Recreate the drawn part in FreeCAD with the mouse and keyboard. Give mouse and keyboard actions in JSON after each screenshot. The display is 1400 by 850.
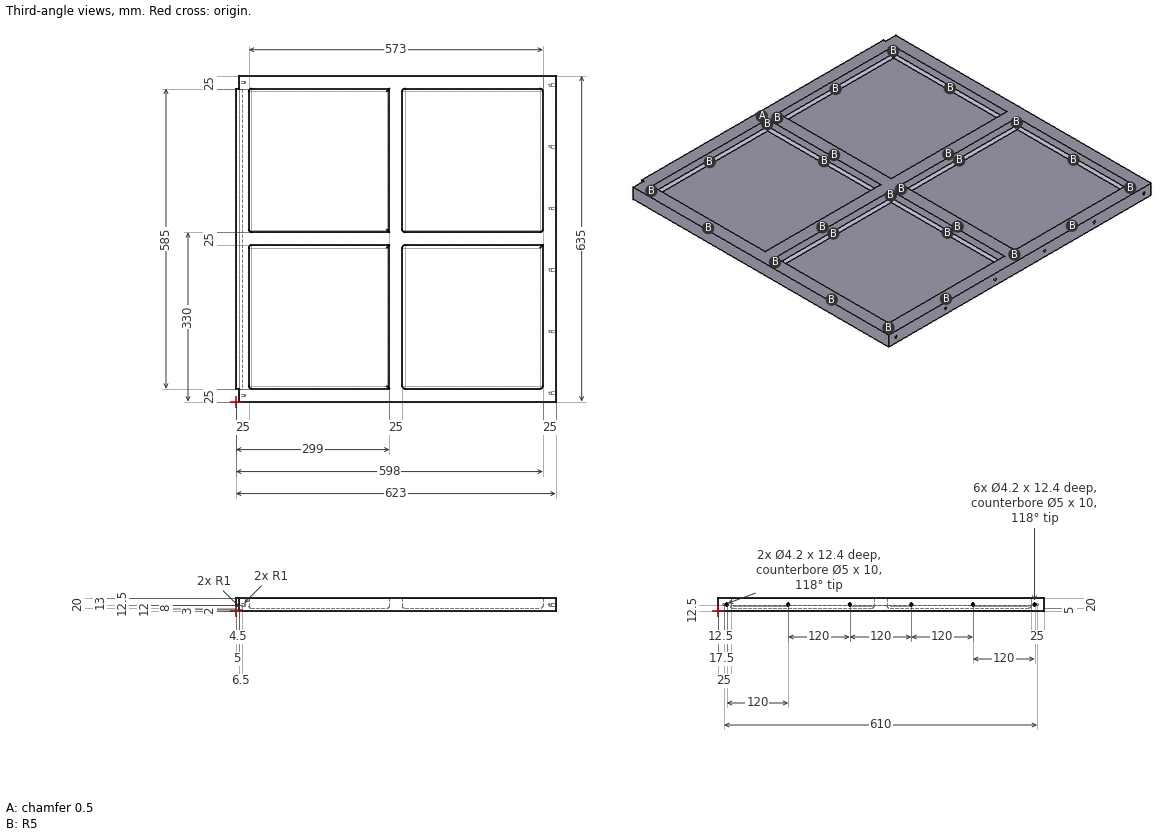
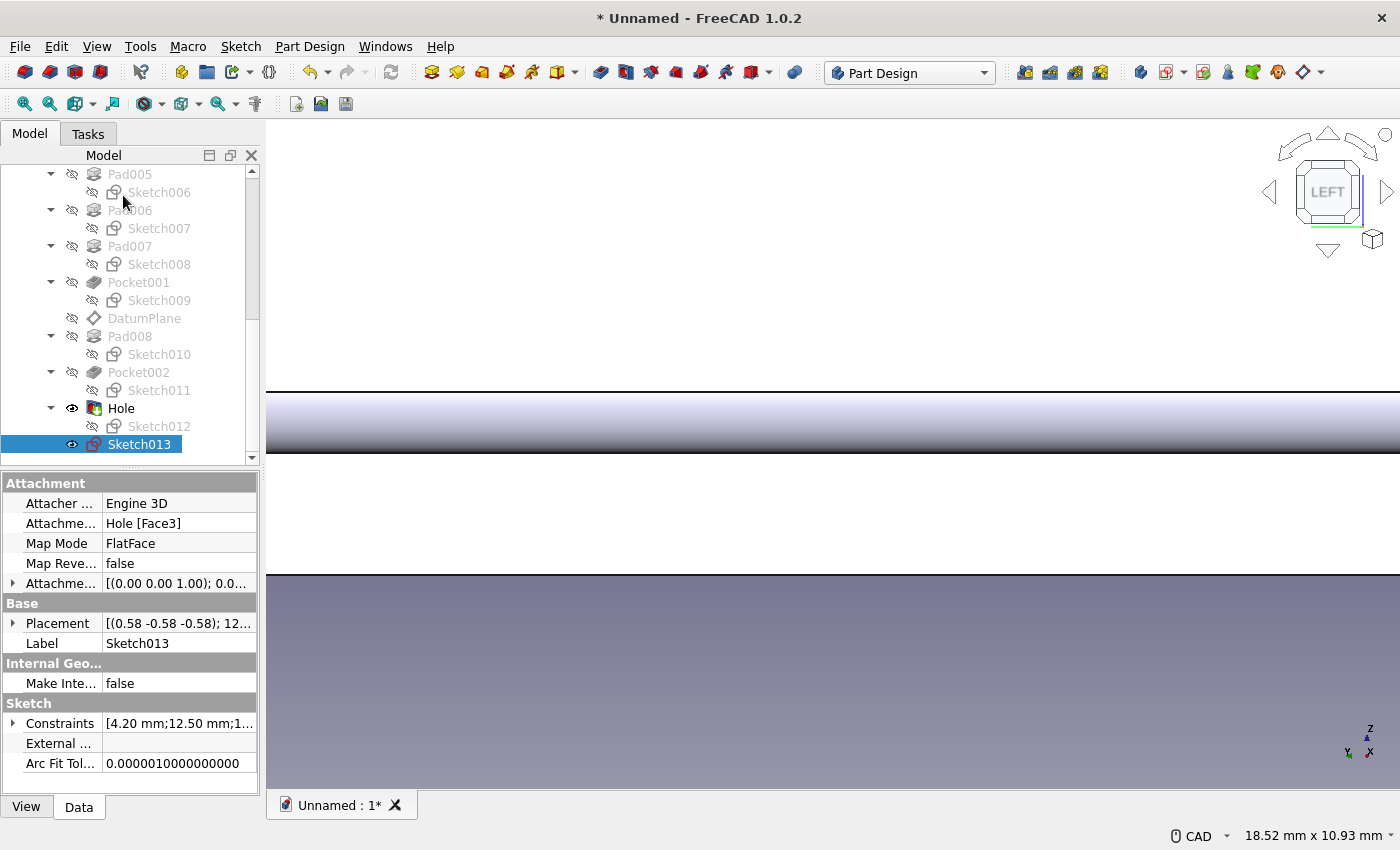
{"action": "left_click", "coordinate": [626, 72]}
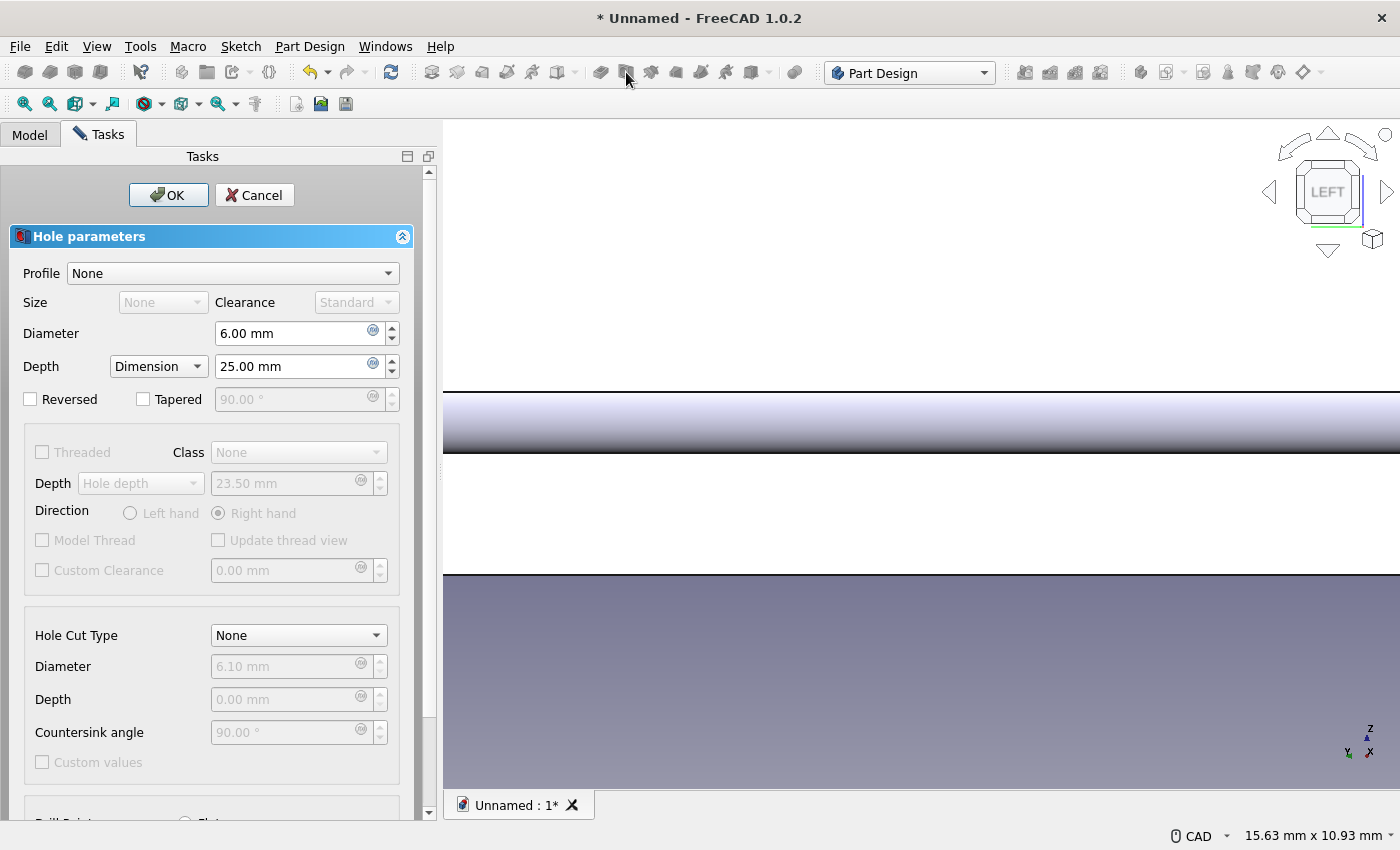
{"action": "triple_click", "coordinate": [300, 334]}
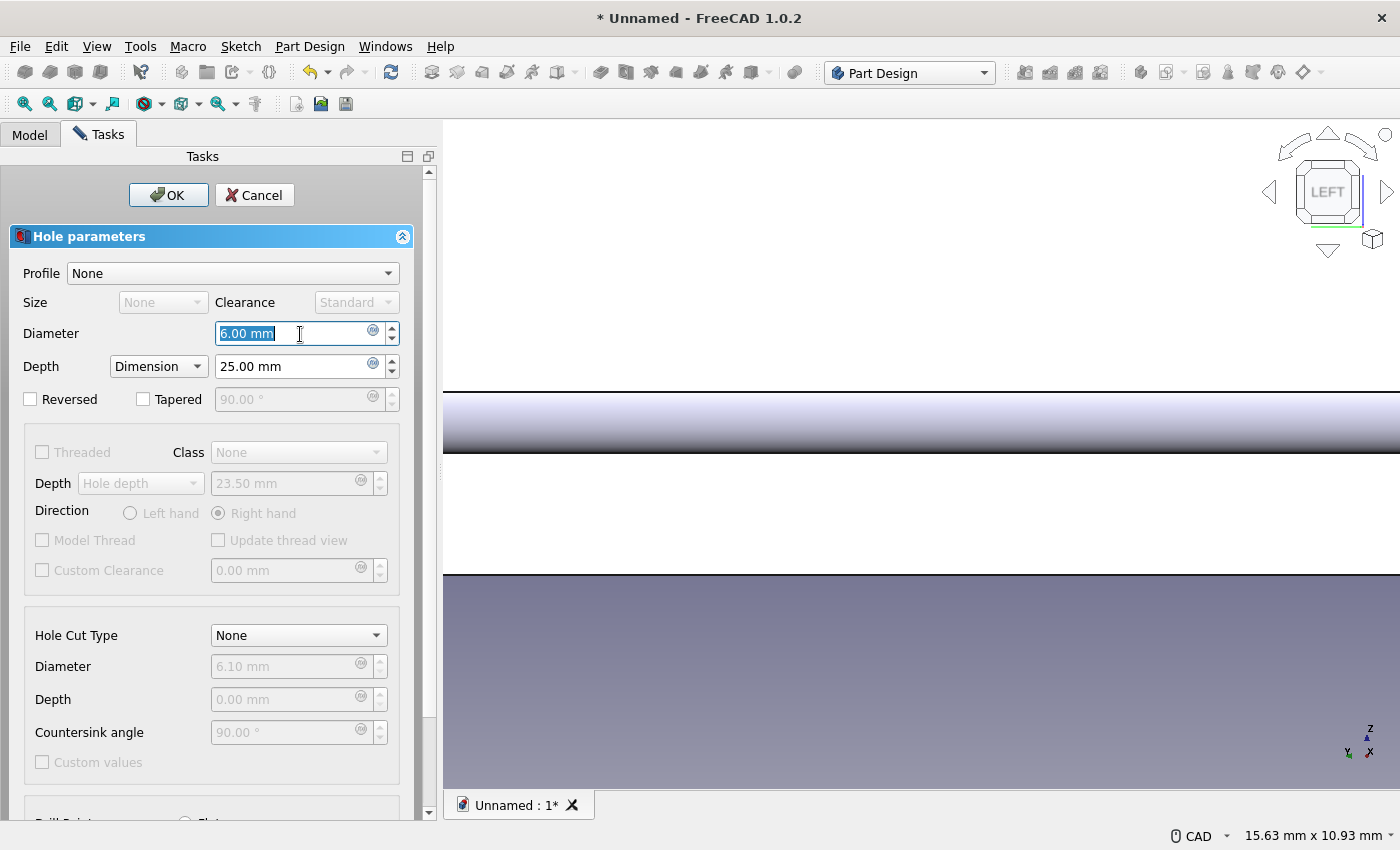
{"action": "type", "text": "4.2"}
{"action": "key", "text": "Tab"}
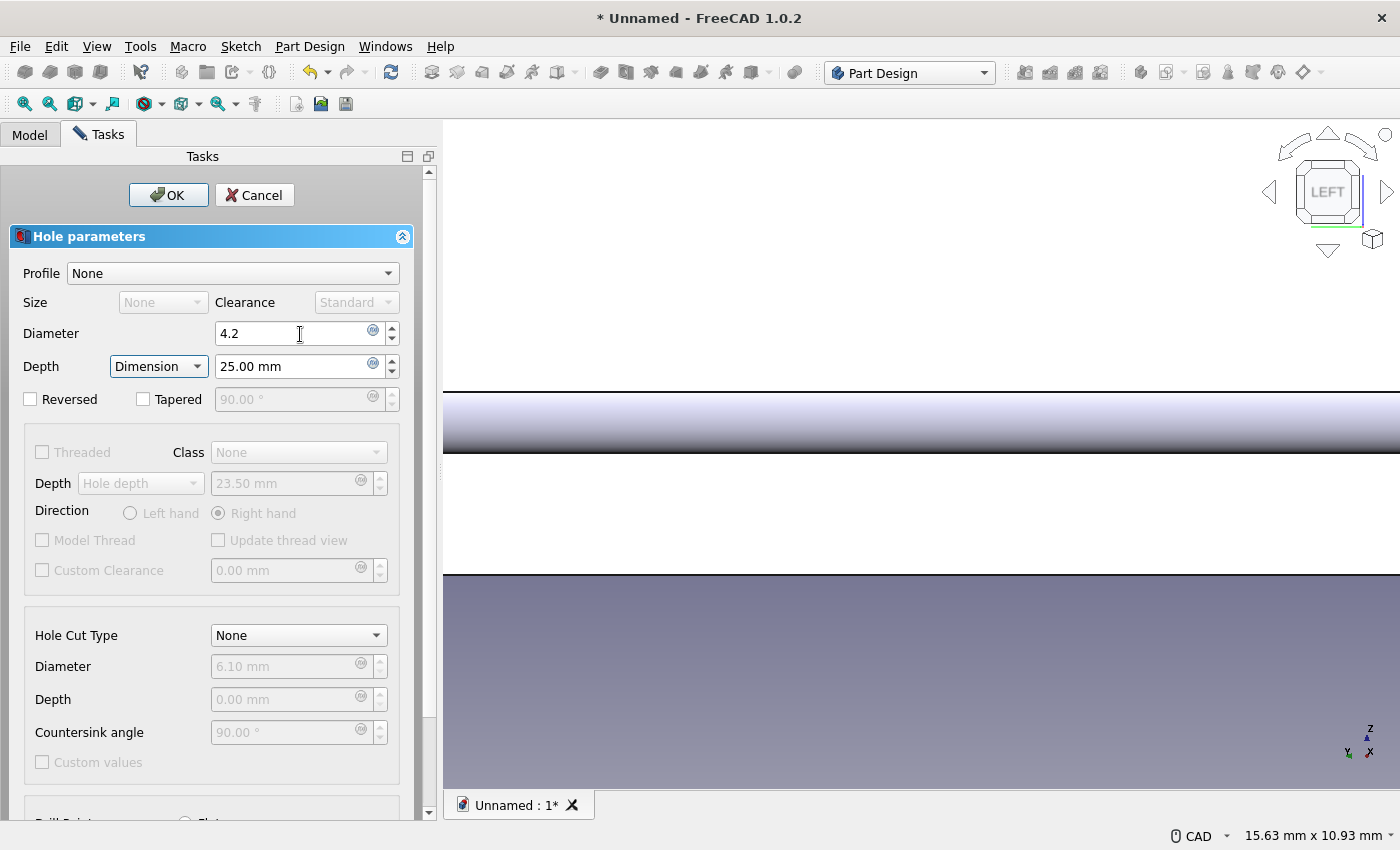
{"action": "triple_click", "coordinate": [300, 366]}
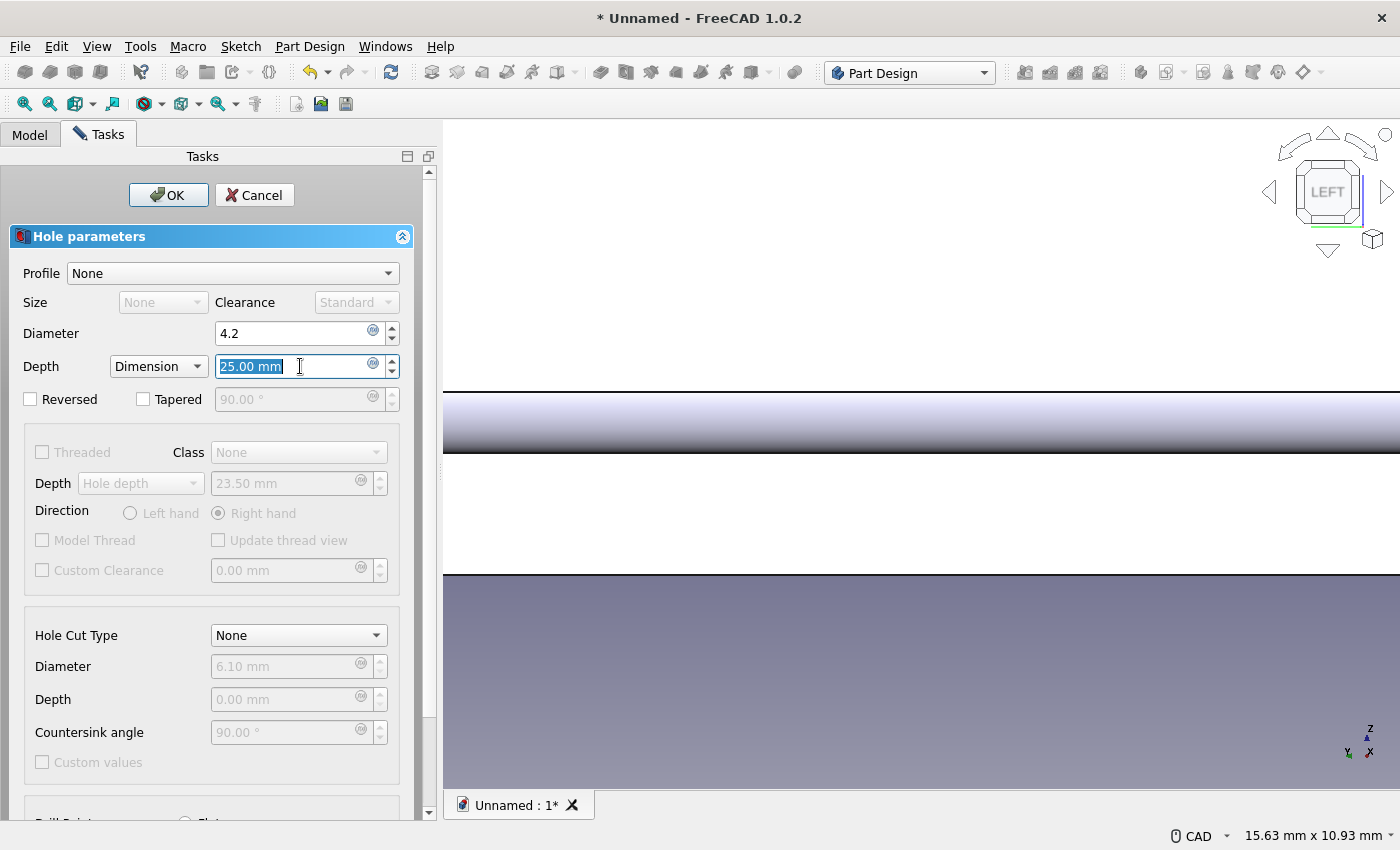
{"action": "type", "text": "12.4"}
{"action": "key", "text": "Tab"}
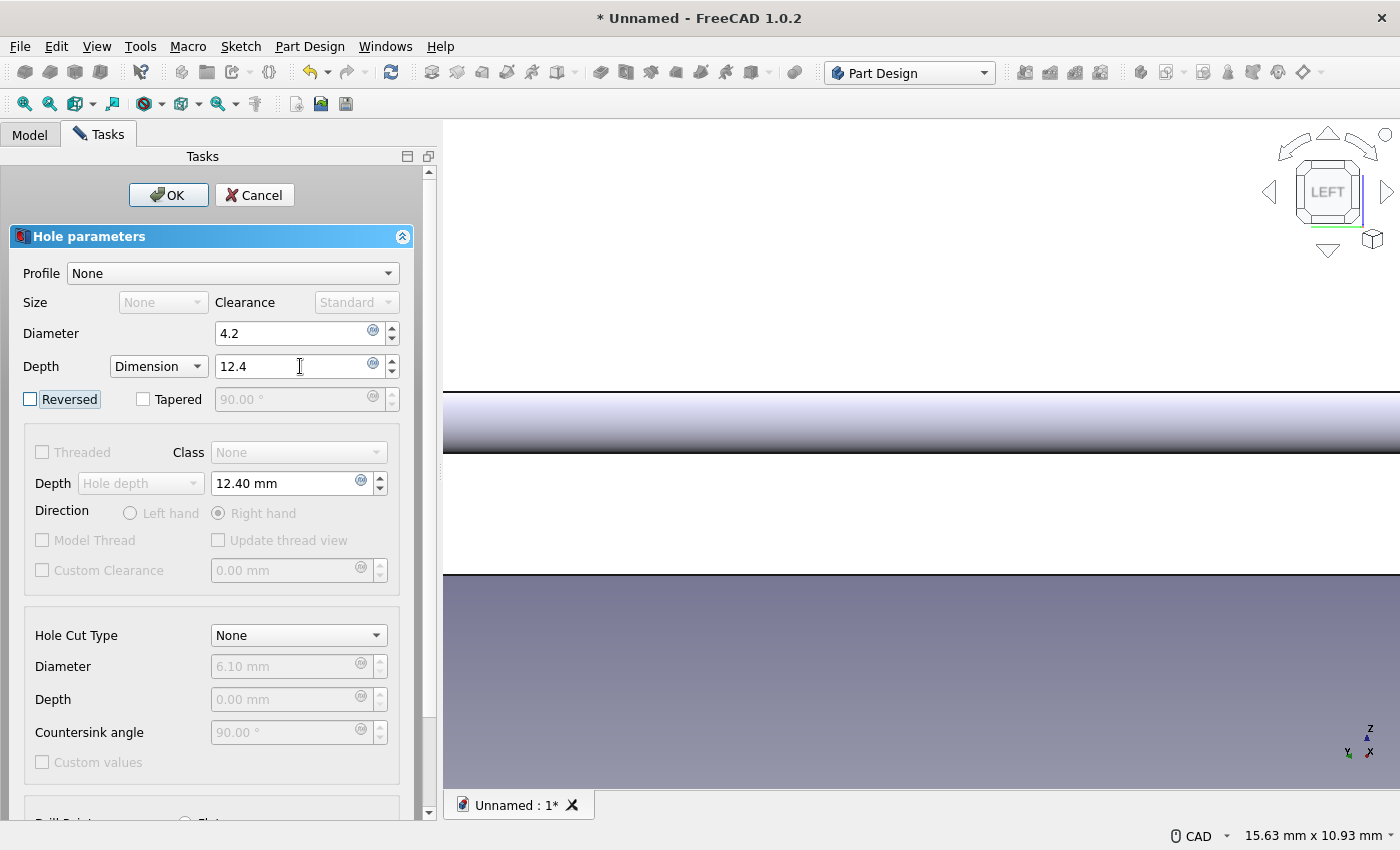
{"action": "left_click", "coordinate": [300, 636]}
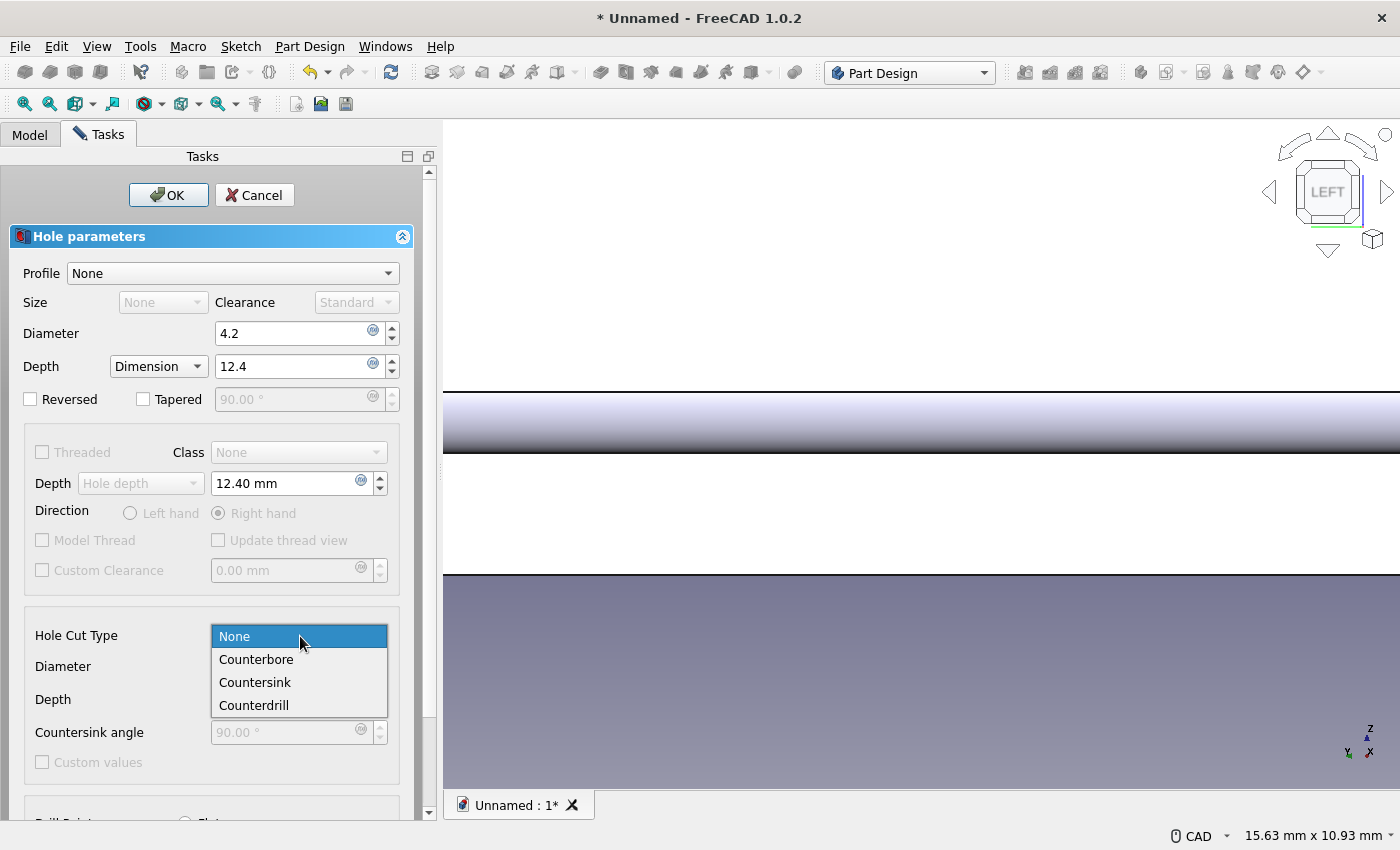
{"action": "left_click", "coordinate": [298, 660]}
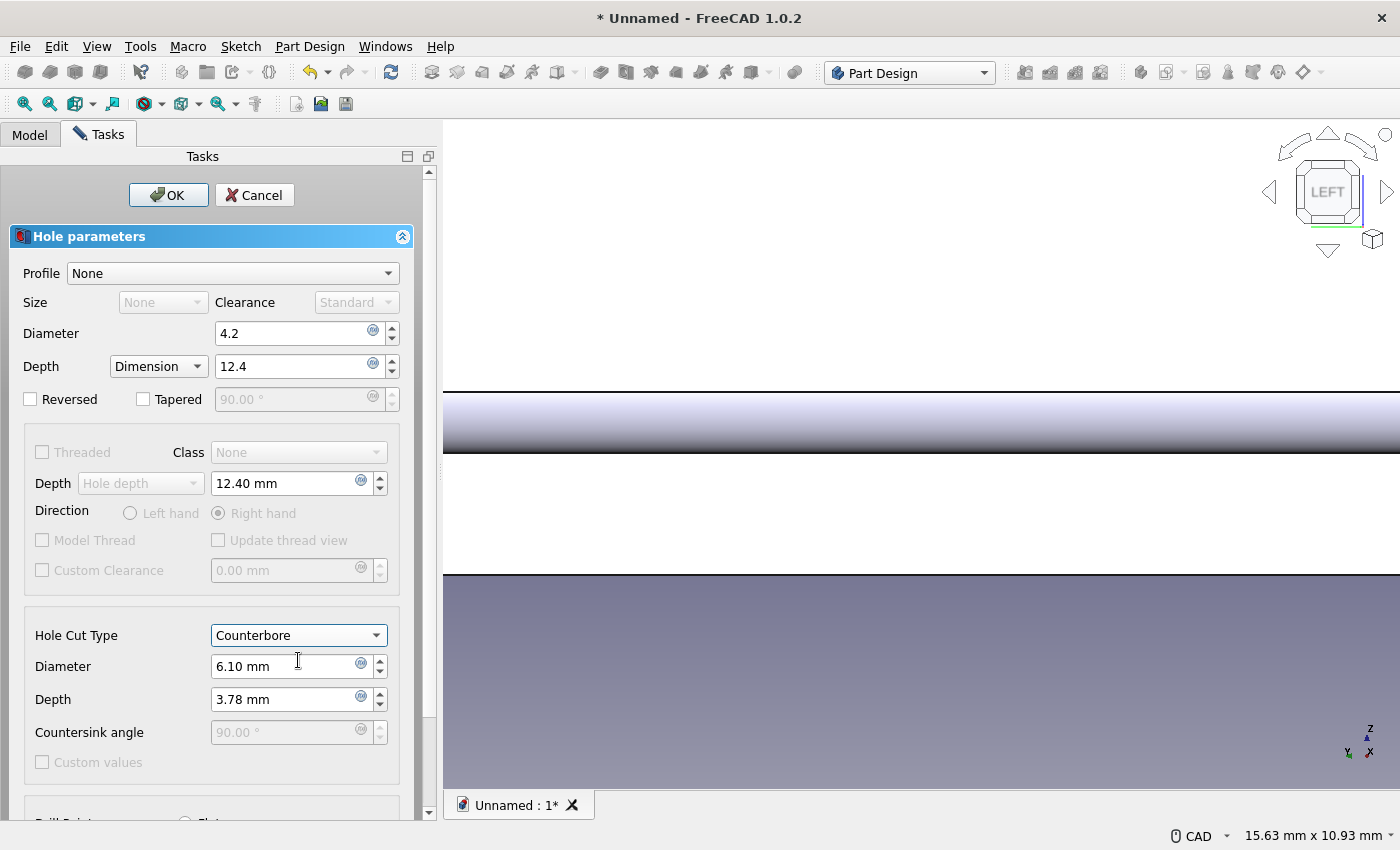
{"action": "triple_click", "coordinate": [292, 666]}